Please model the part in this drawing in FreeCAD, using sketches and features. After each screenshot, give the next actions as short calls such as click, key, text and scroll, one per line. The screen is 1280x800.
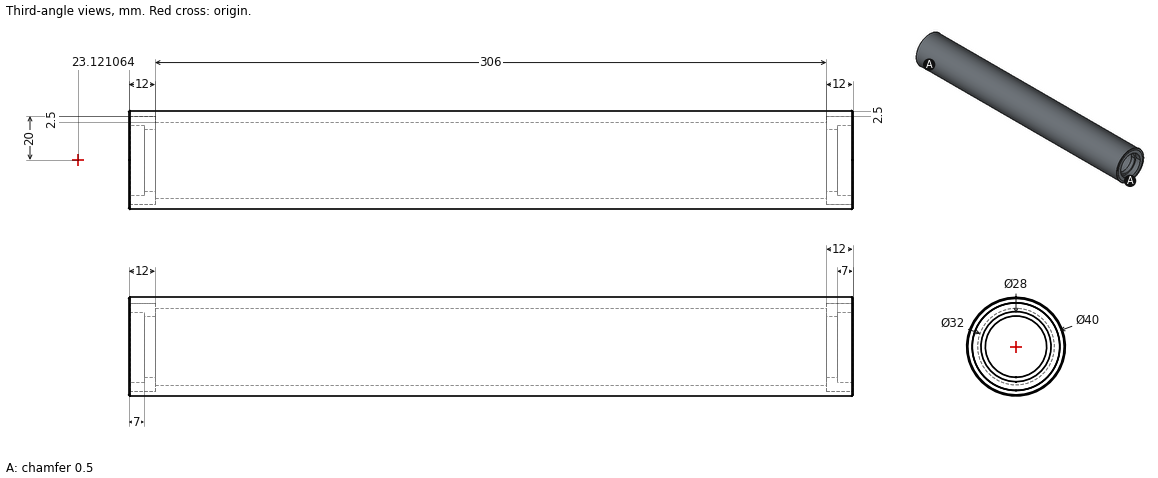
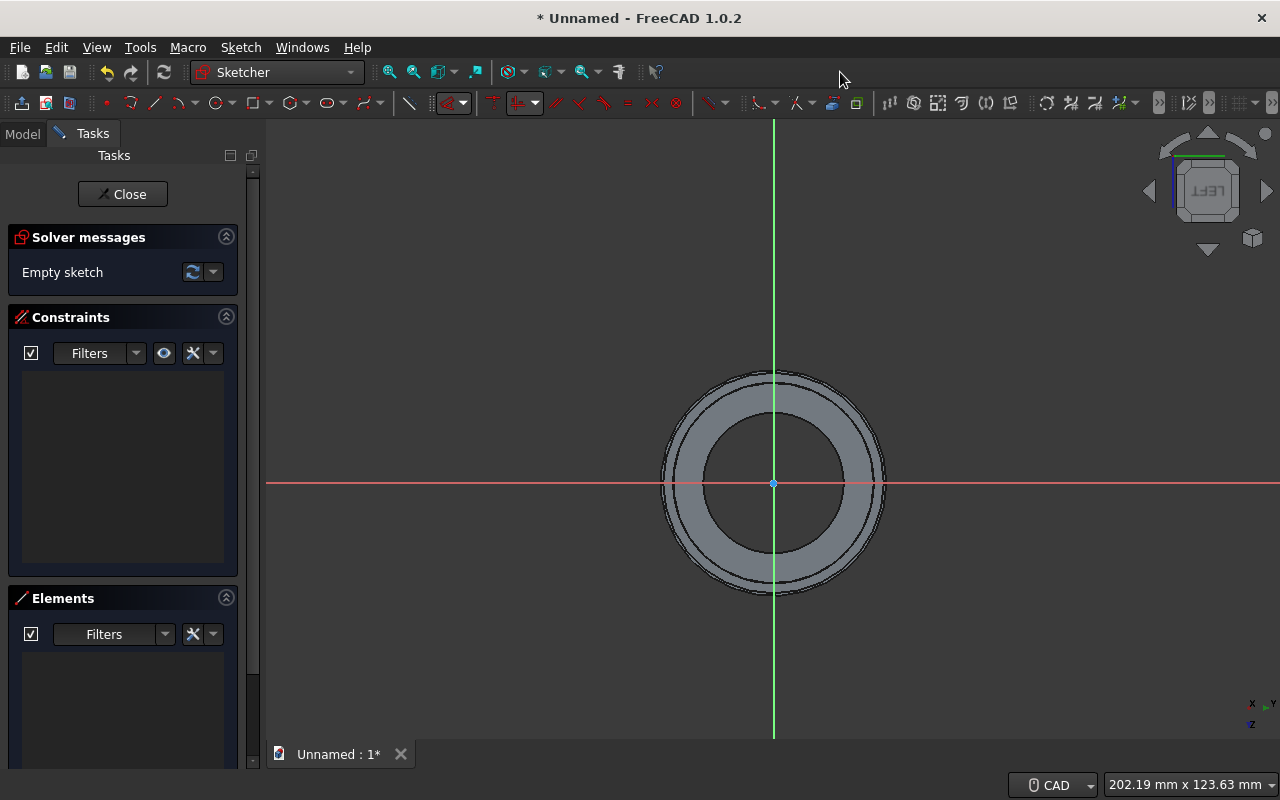
scroll(814, 514, up, 5)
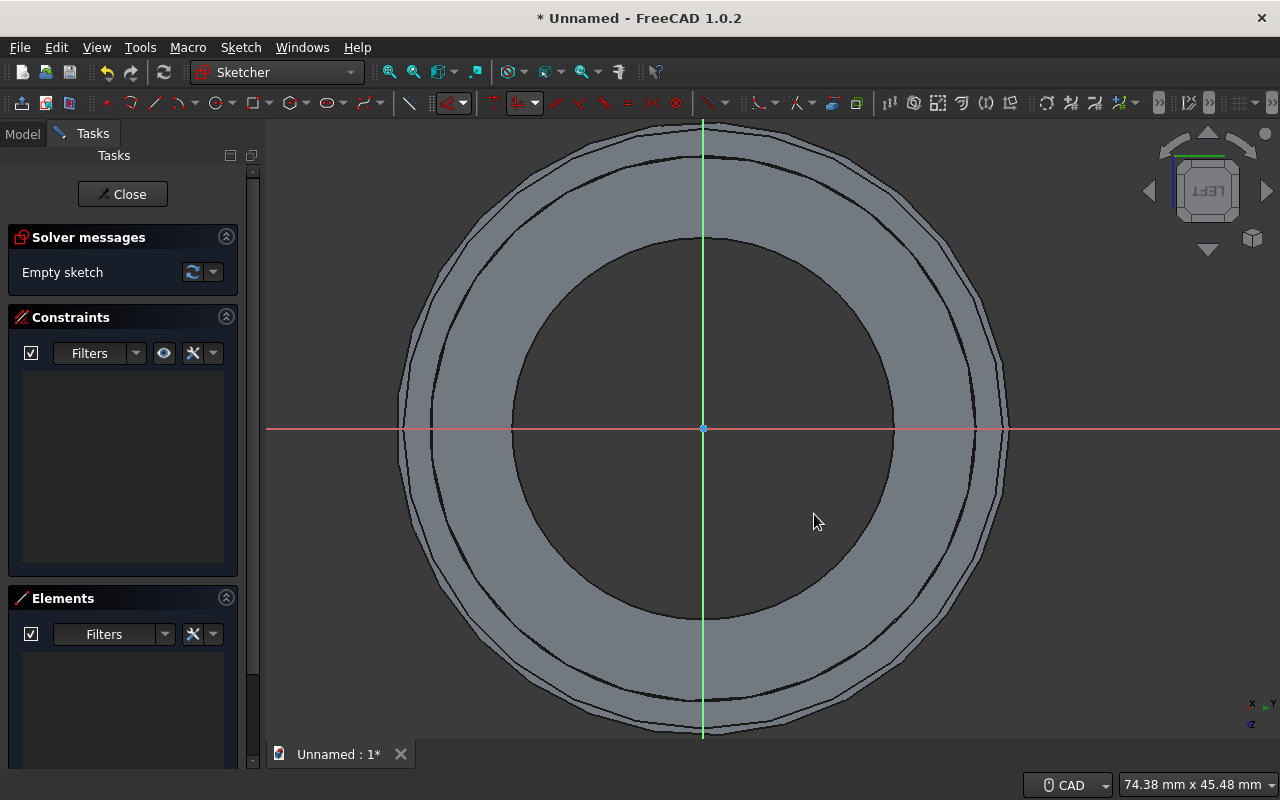
click(216, 104)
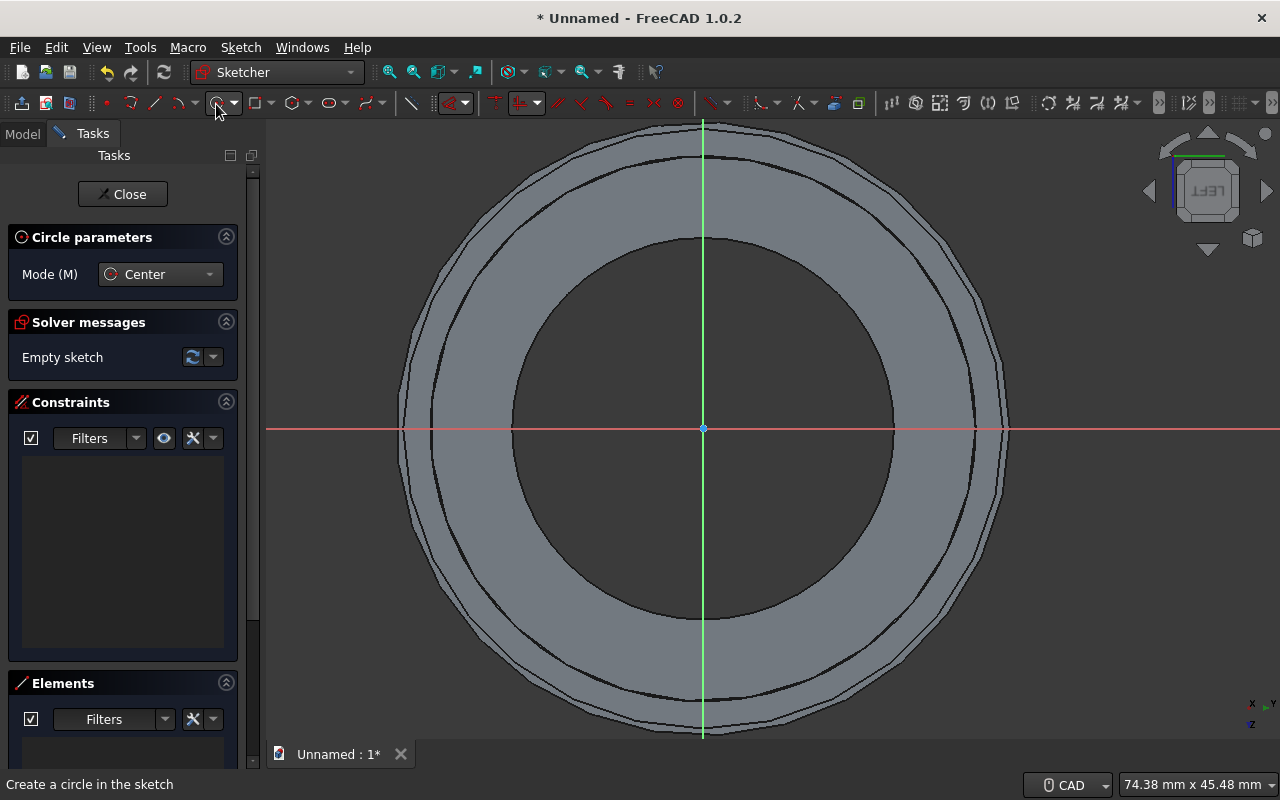
click(703, 429)
move(857, 275)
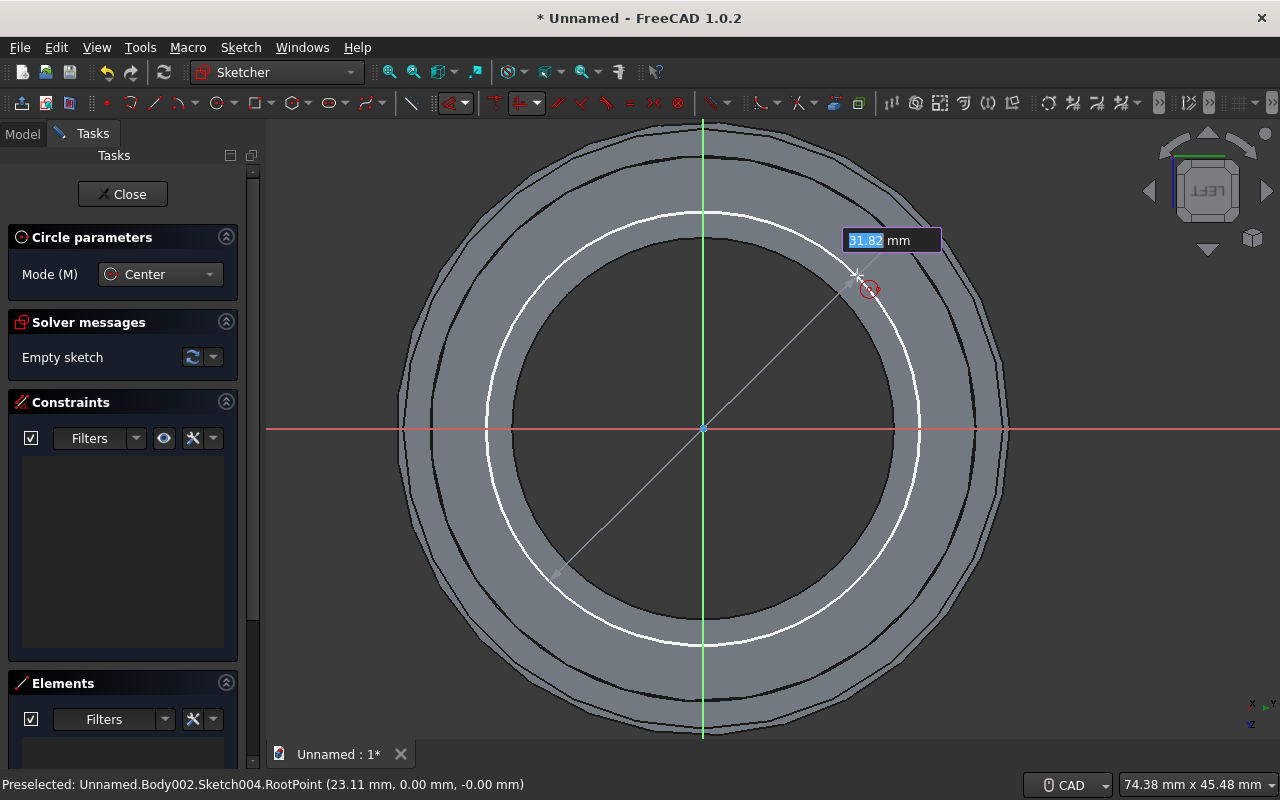
text(32)
key(Return)
key(Escape)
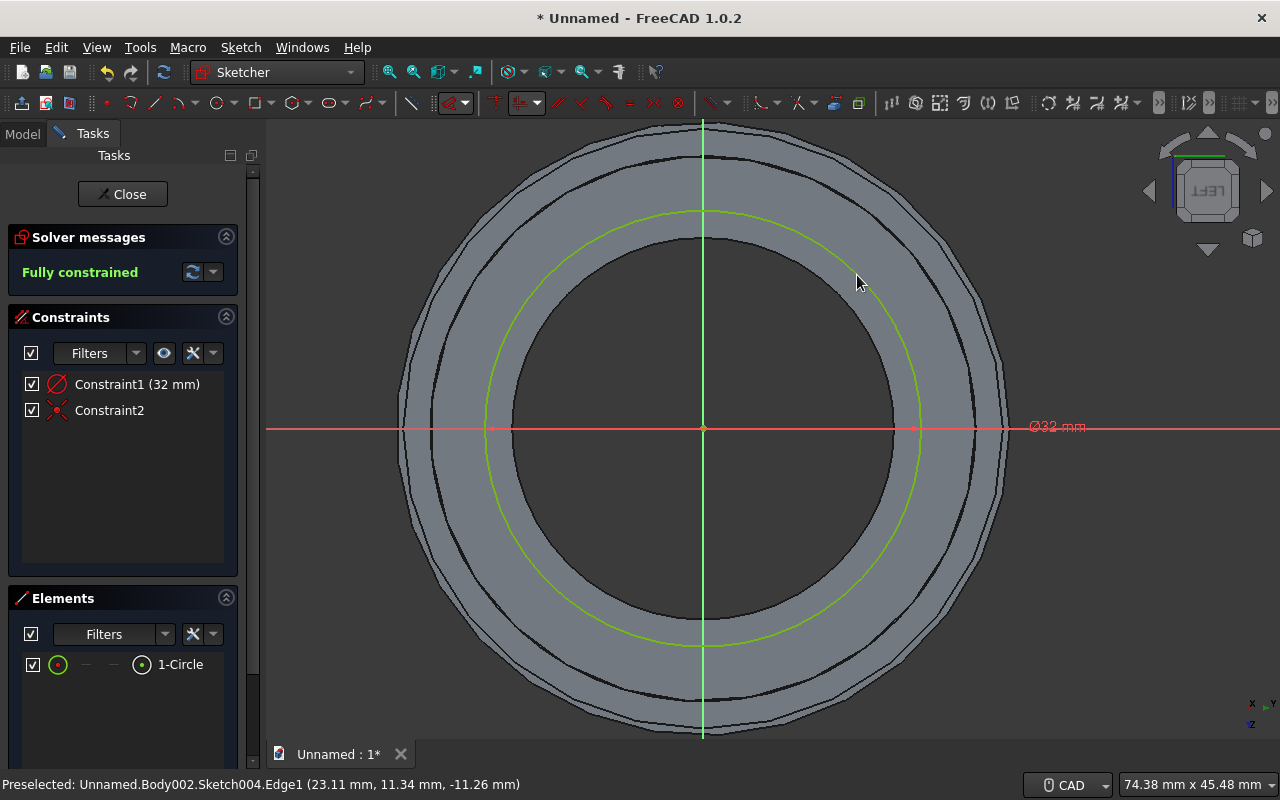
click(123, 194)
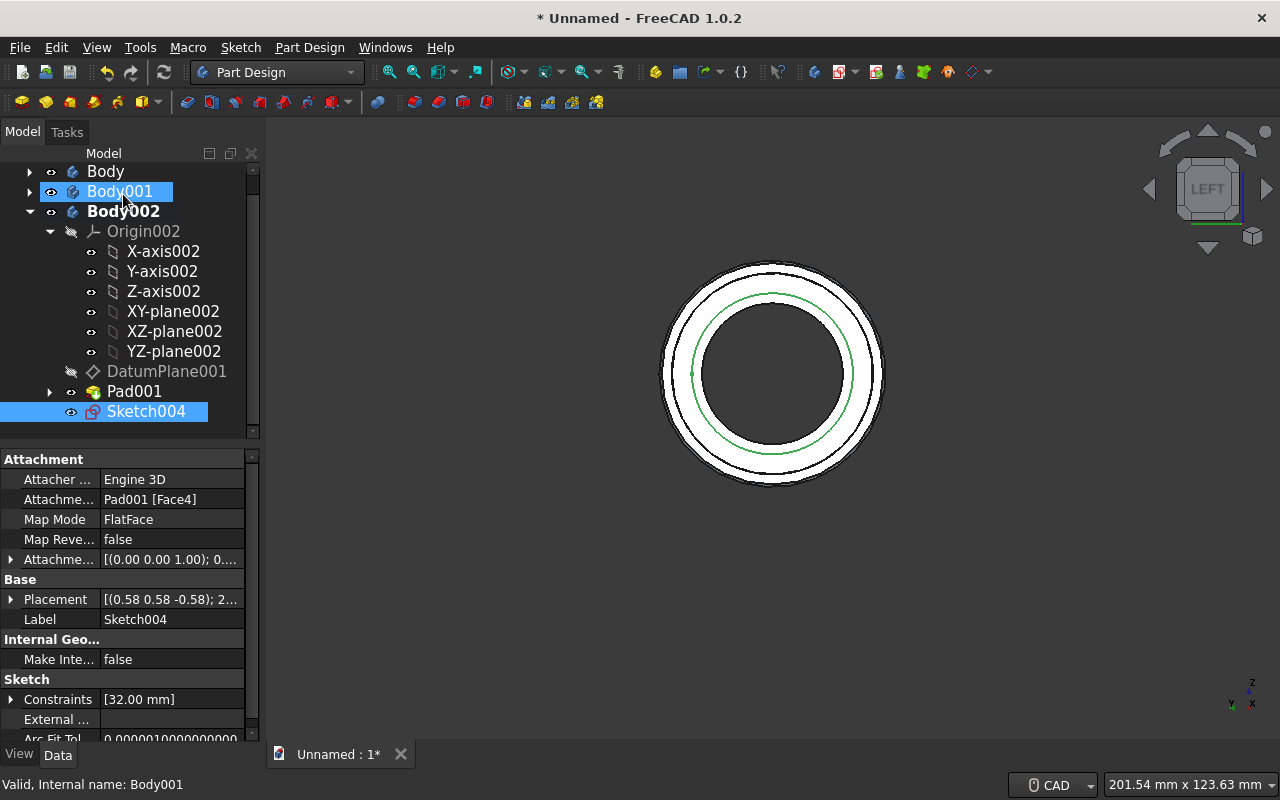
click(188, 102)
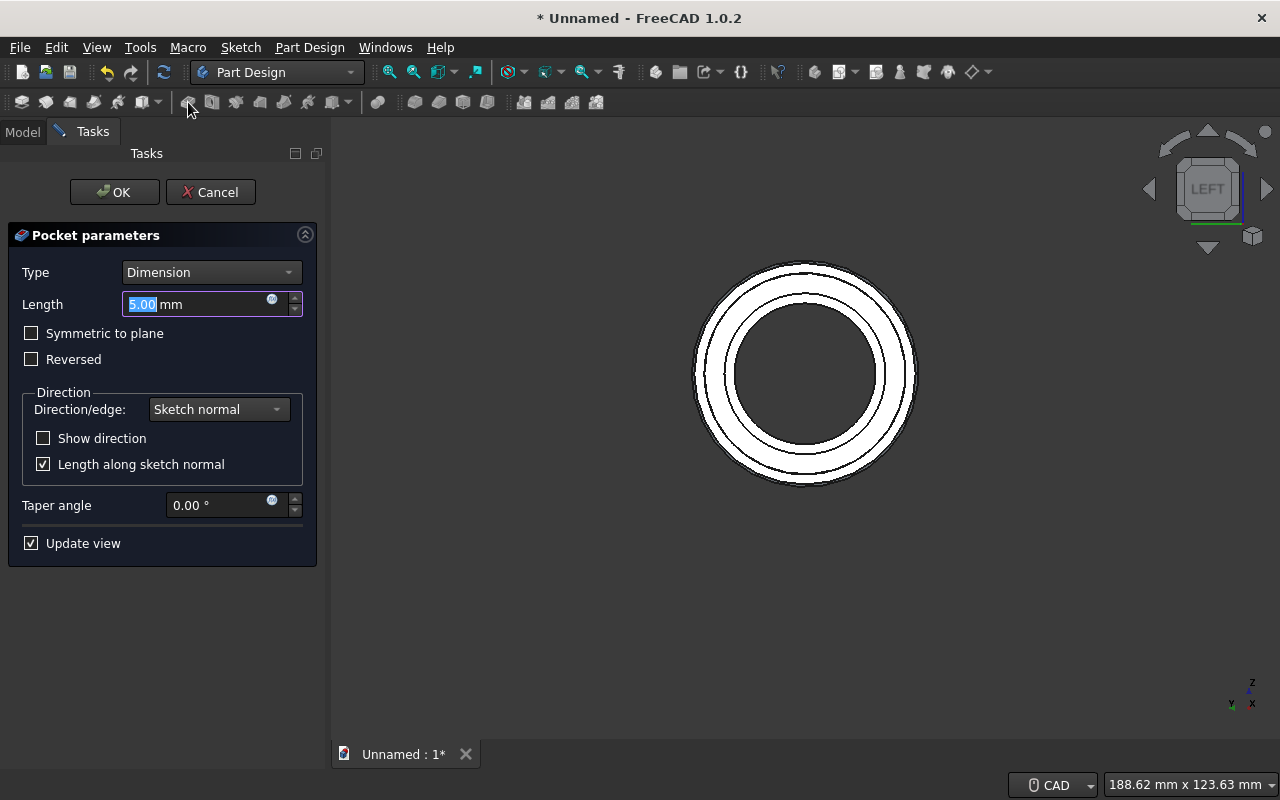
text(7)
key(Tab)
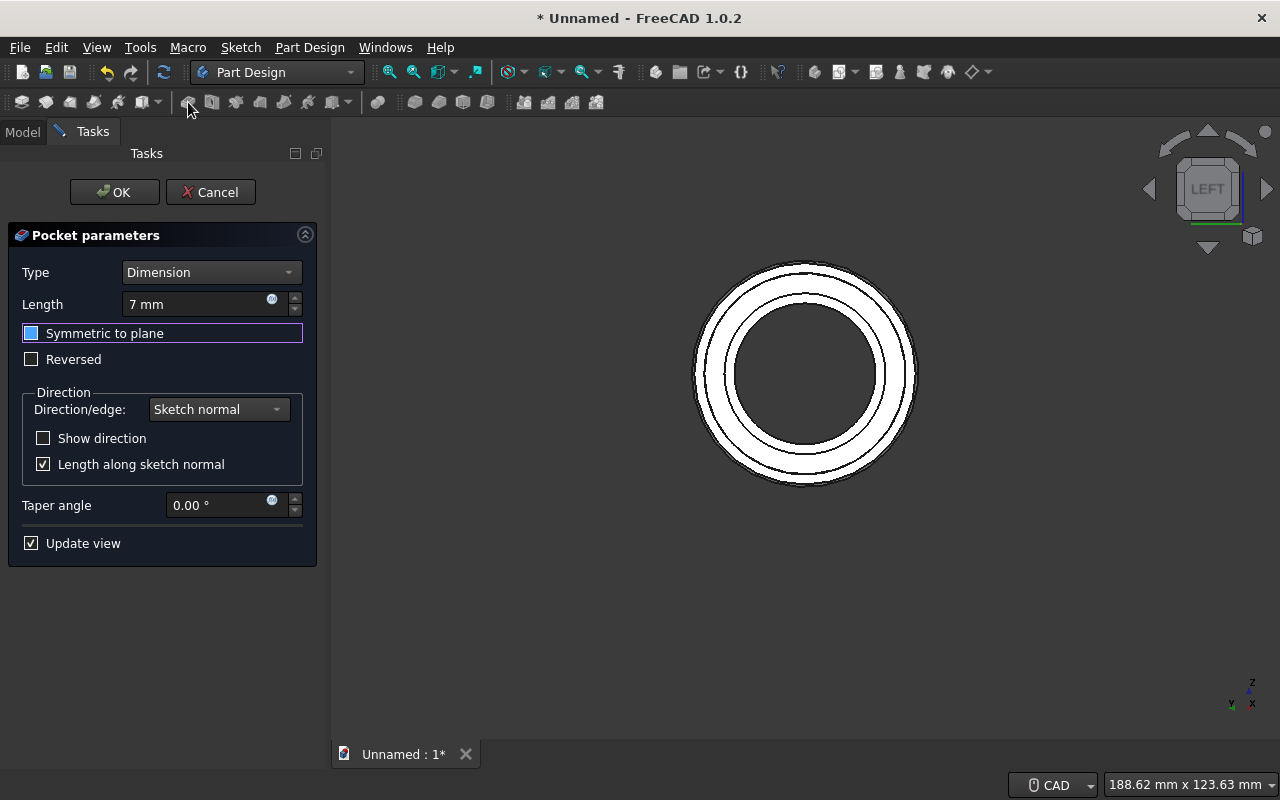
click(115, 192)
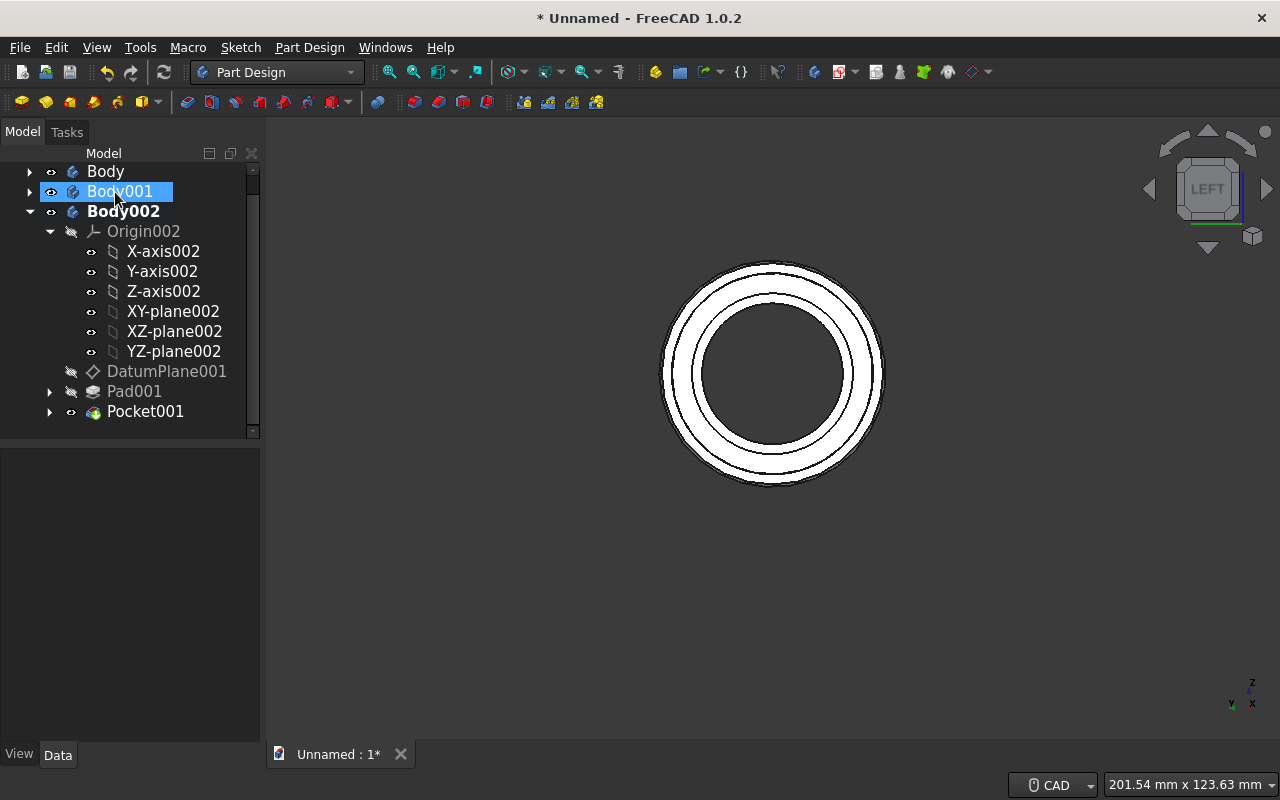
key(0)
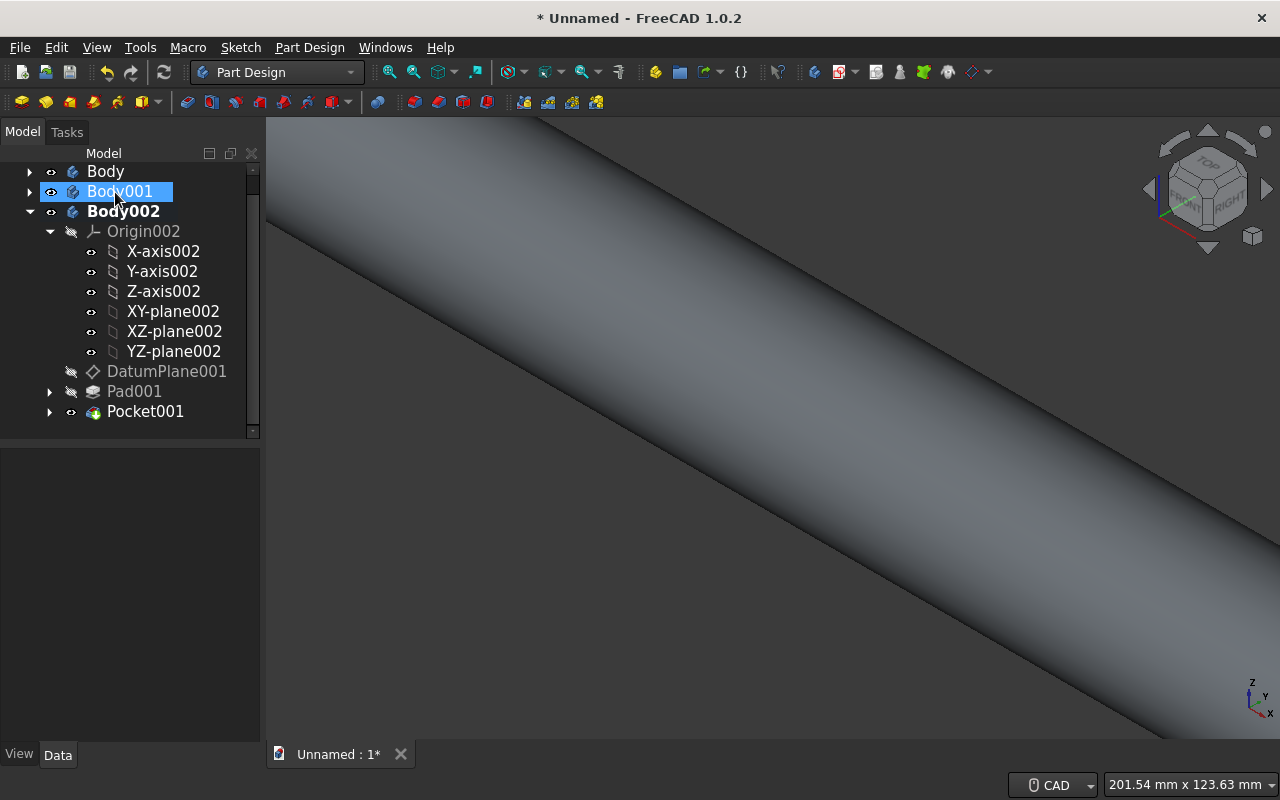
click(390, 72)